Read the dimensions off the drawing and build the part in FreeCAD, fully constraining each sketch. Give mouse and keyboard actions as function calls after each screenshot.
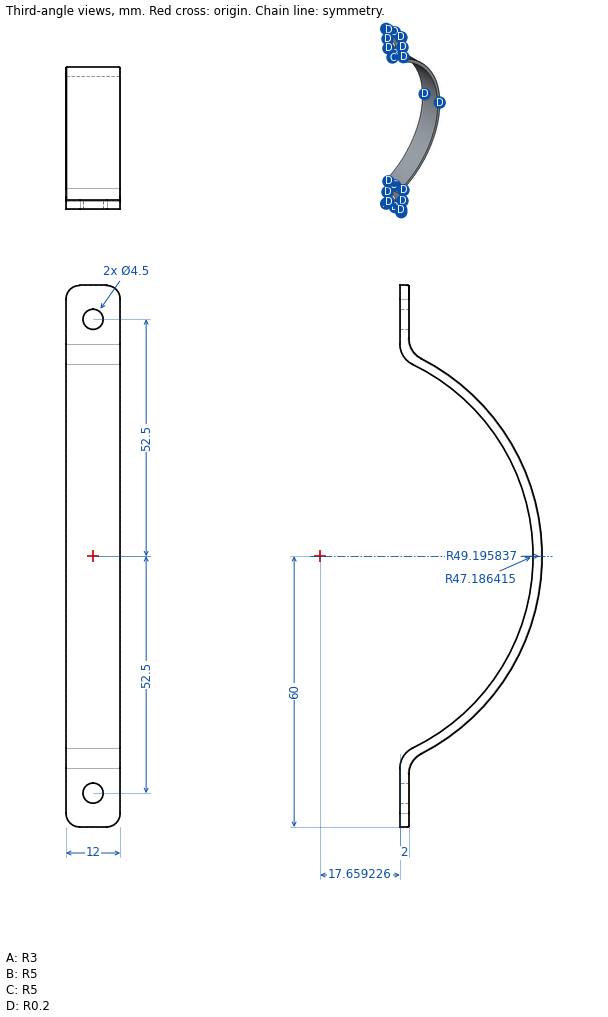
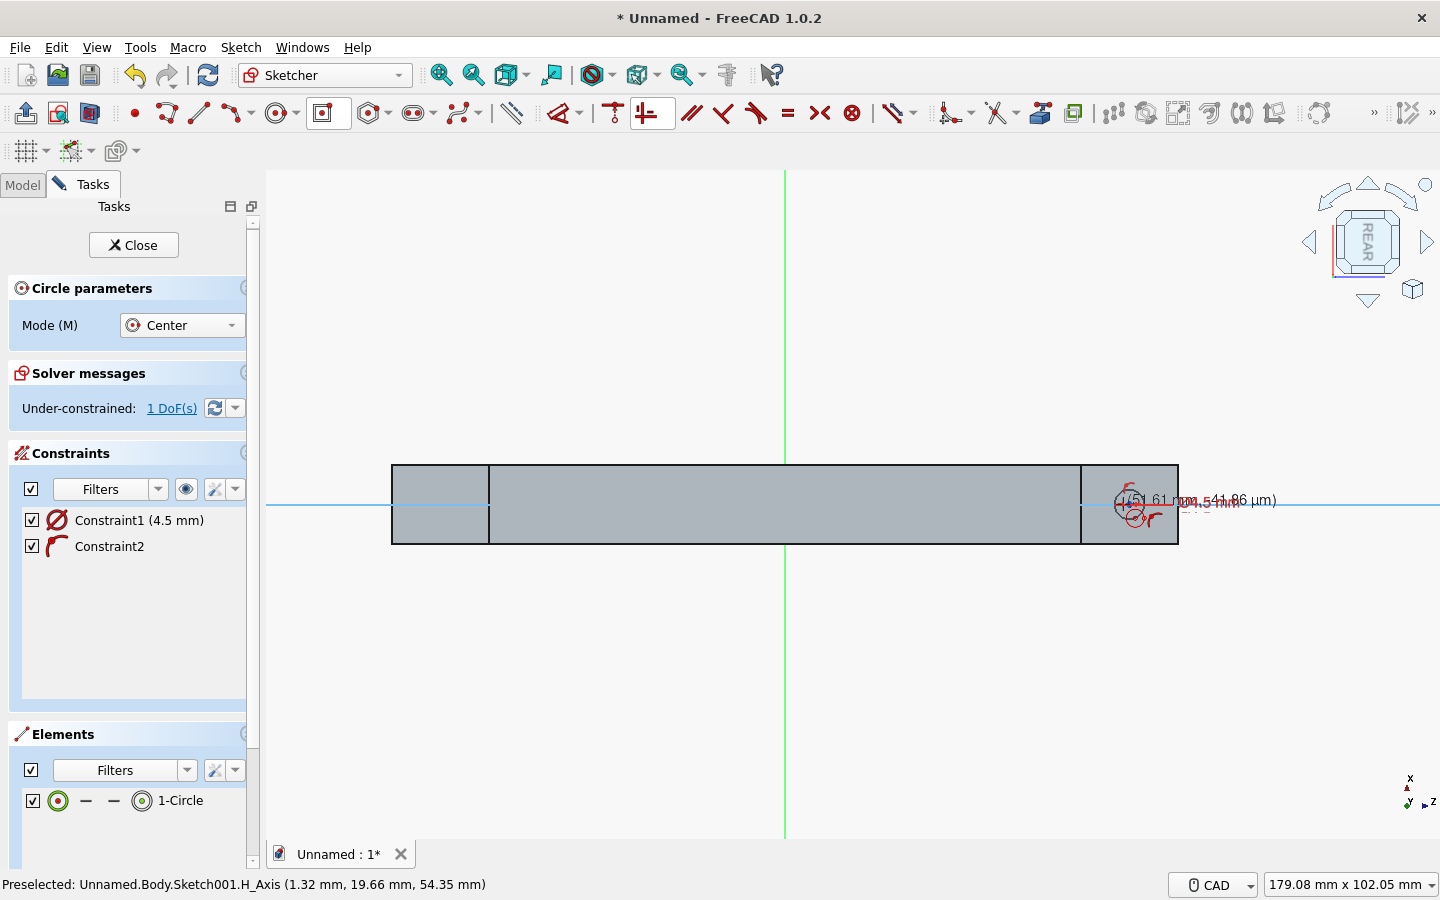
scroll(441, 504, up, 3)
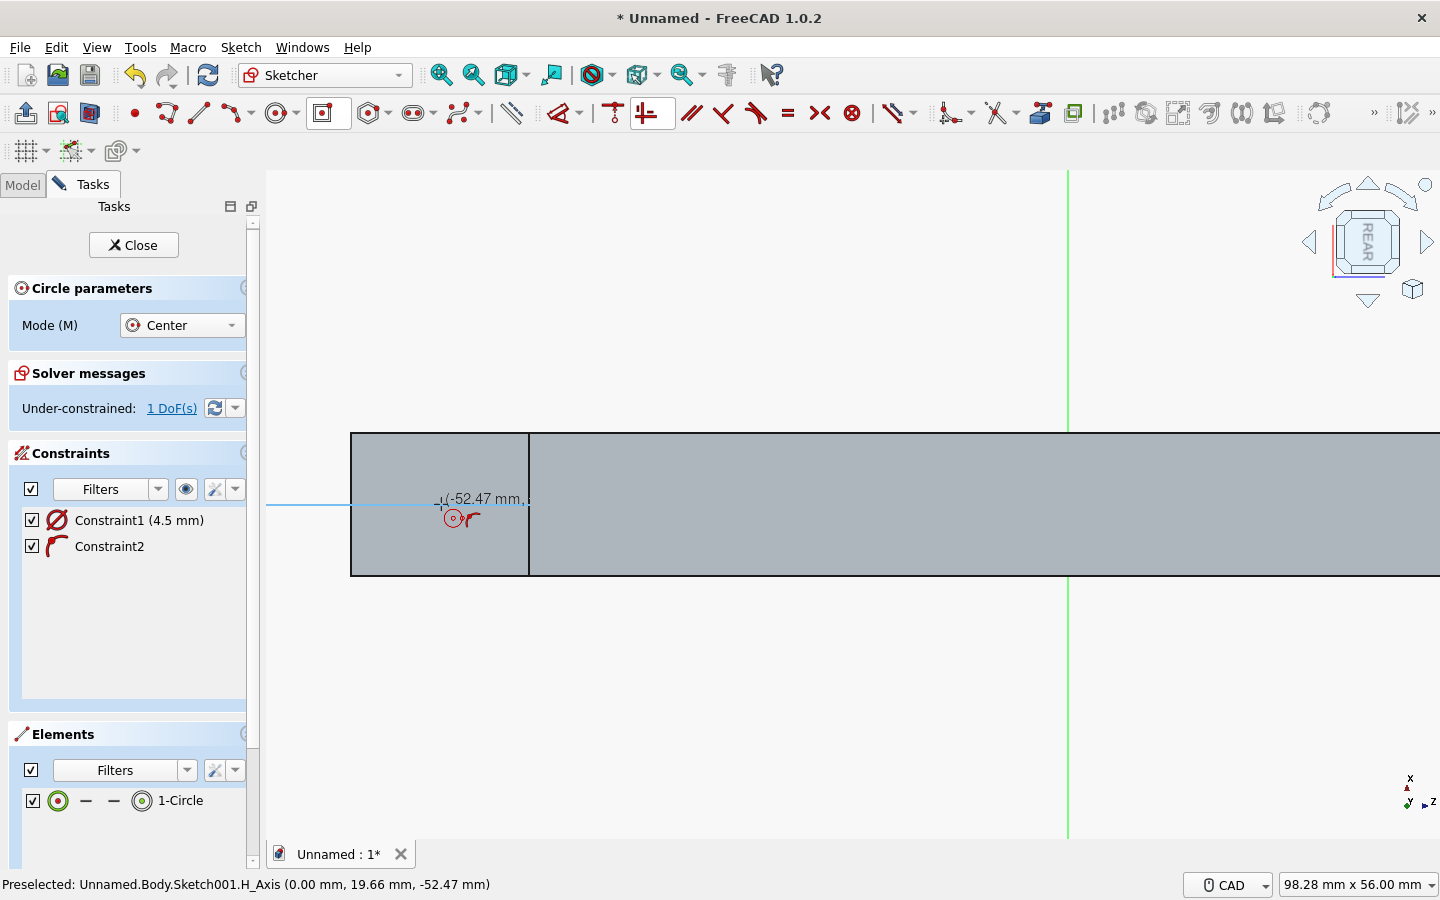
click(441, 504)
move(460, 485)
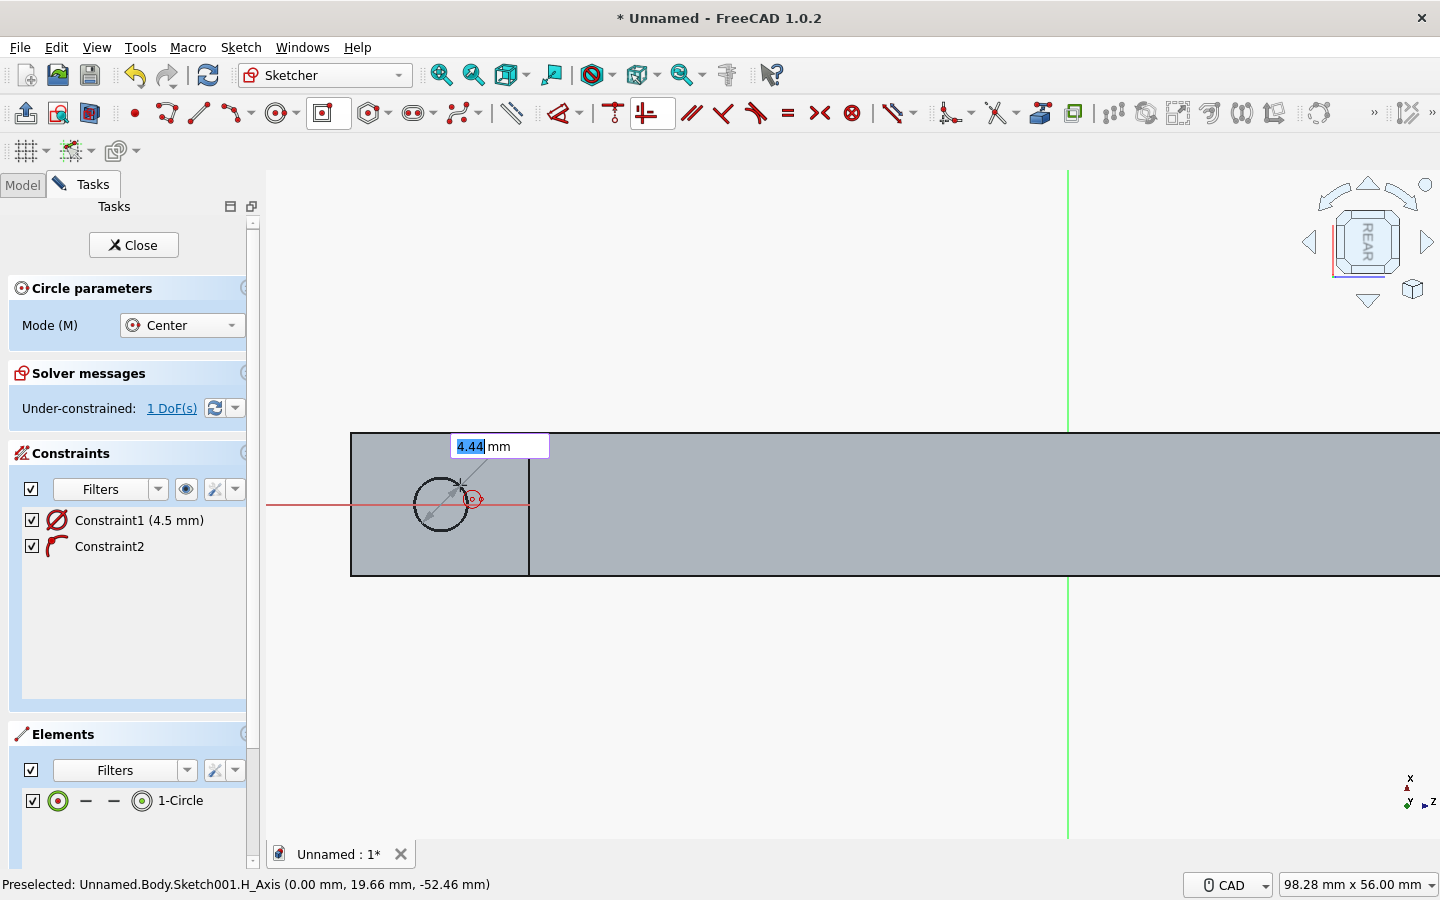
text(4.5)
key(Return)
key(Escape)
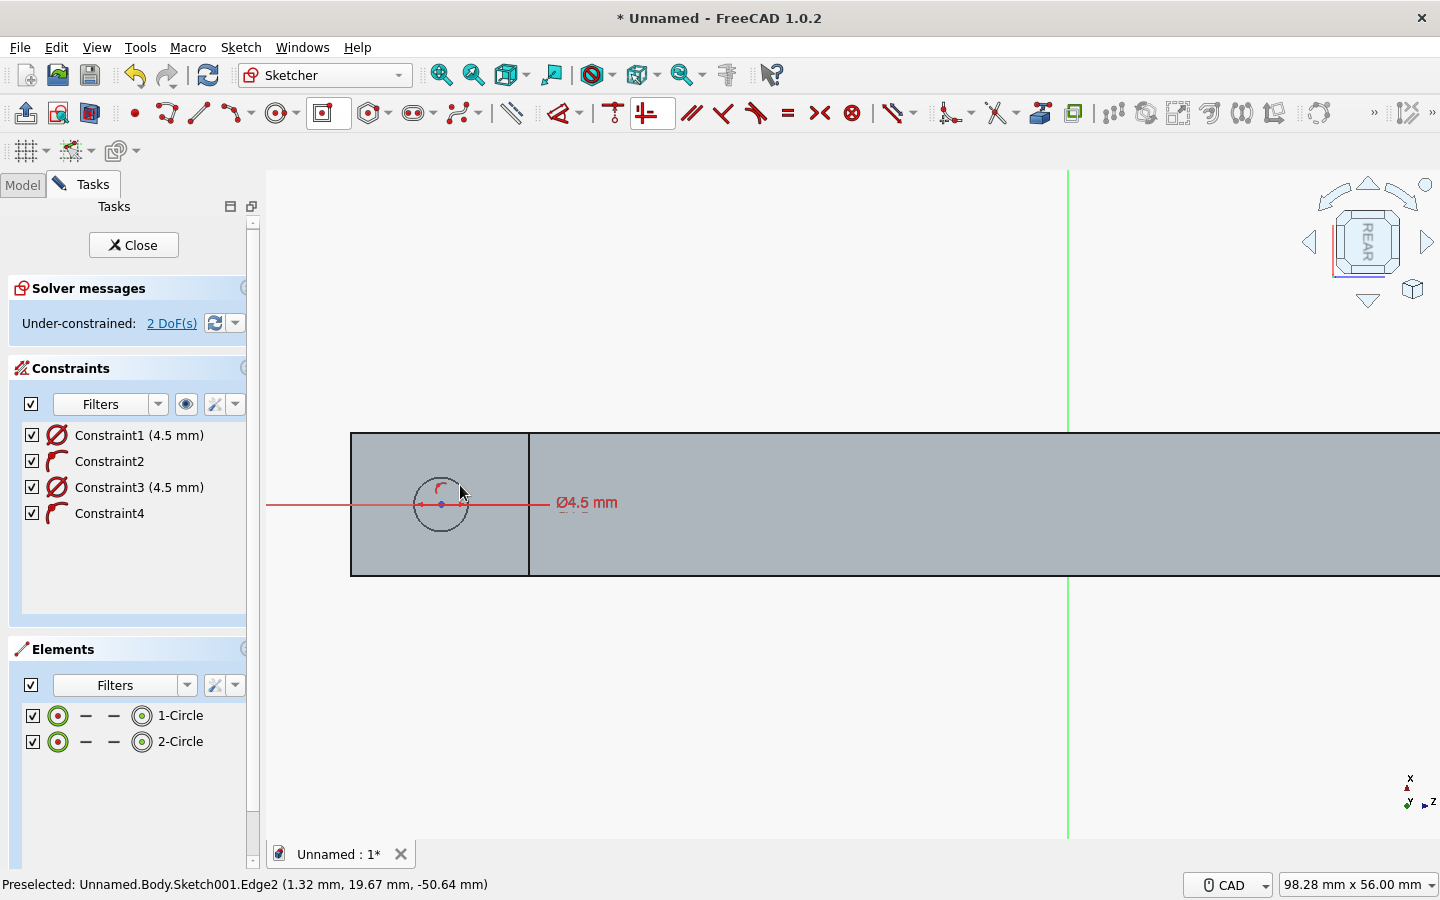
click(558, 114)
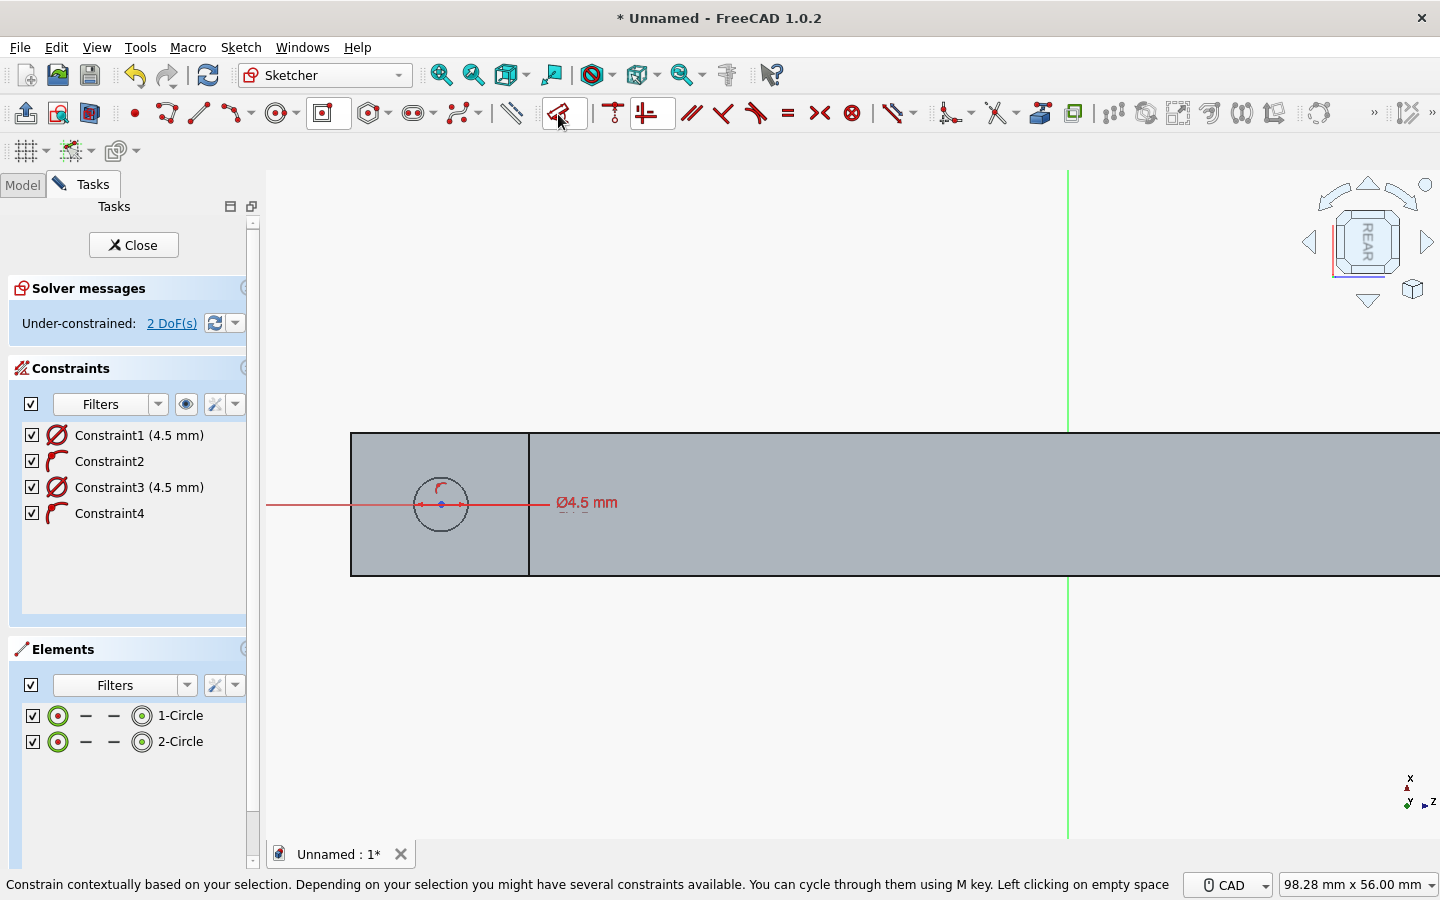
scroll(440, 505, down, 3)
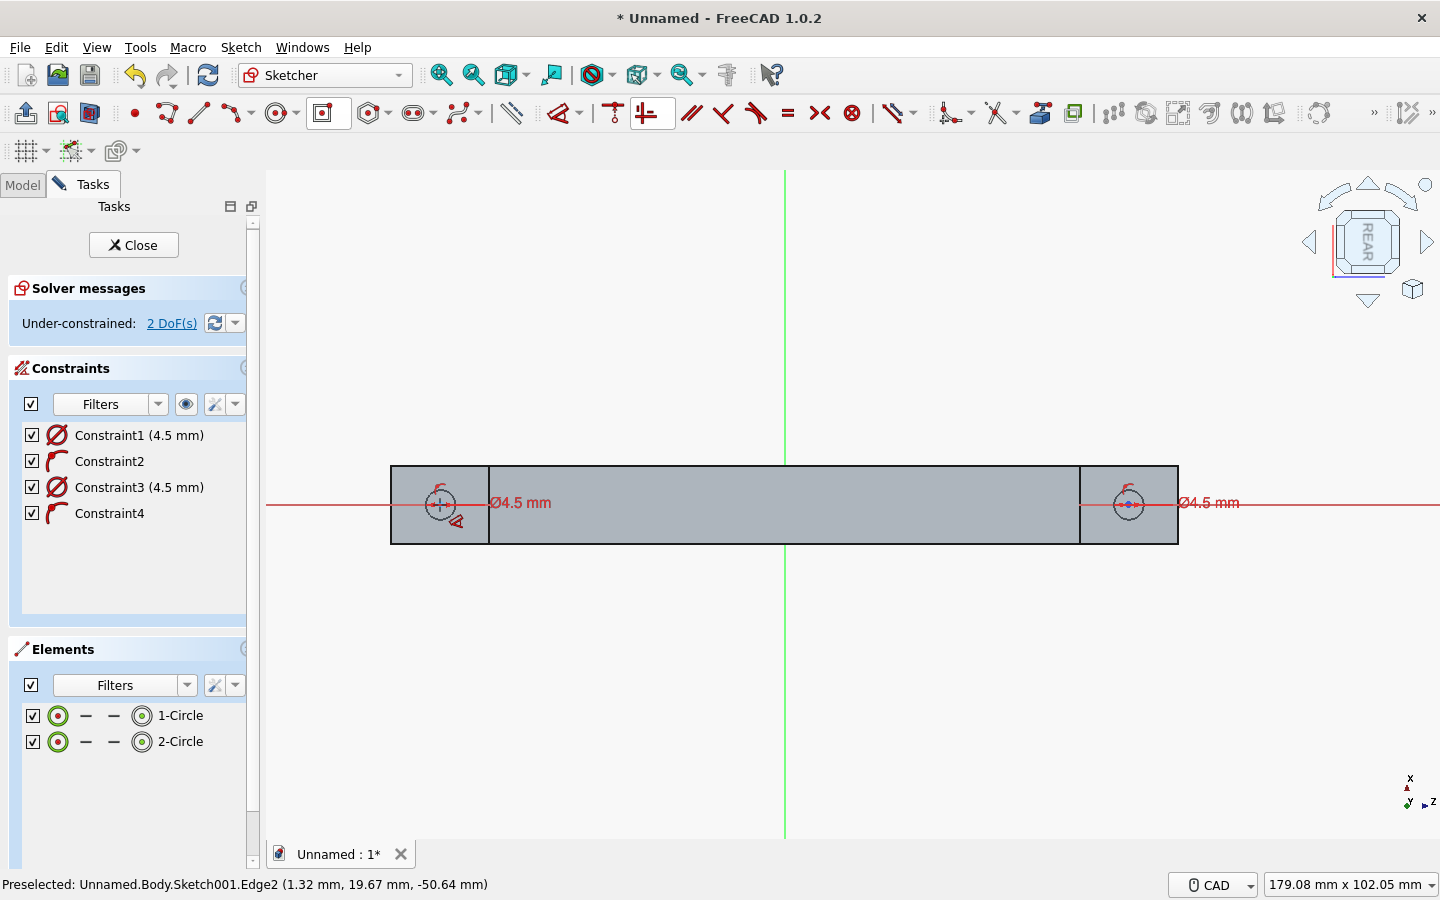
click(1129, 505)
click(957, 539)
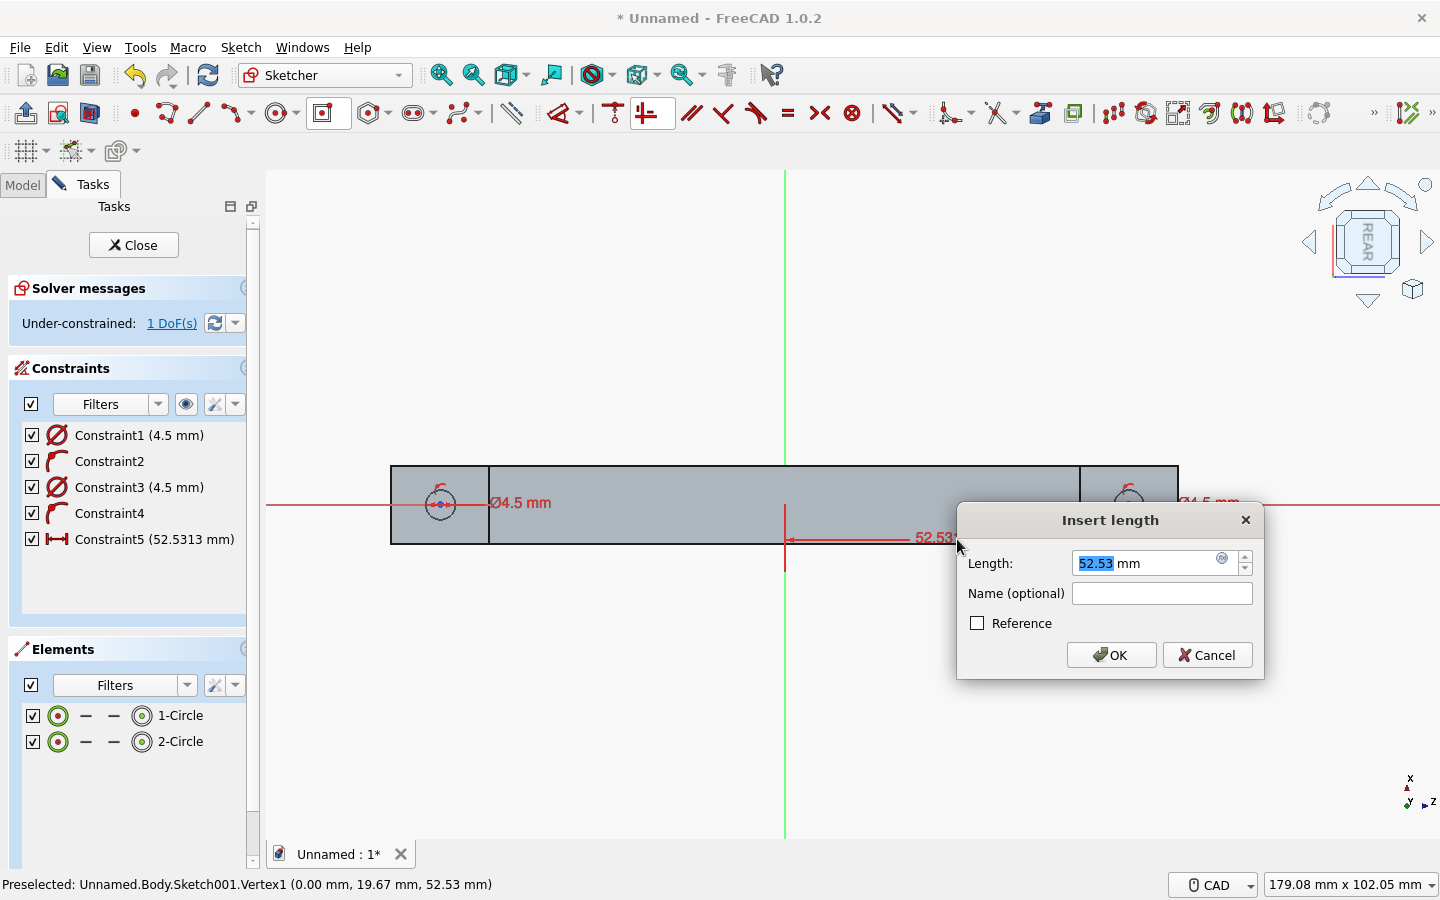
text(52.5)
key(Return)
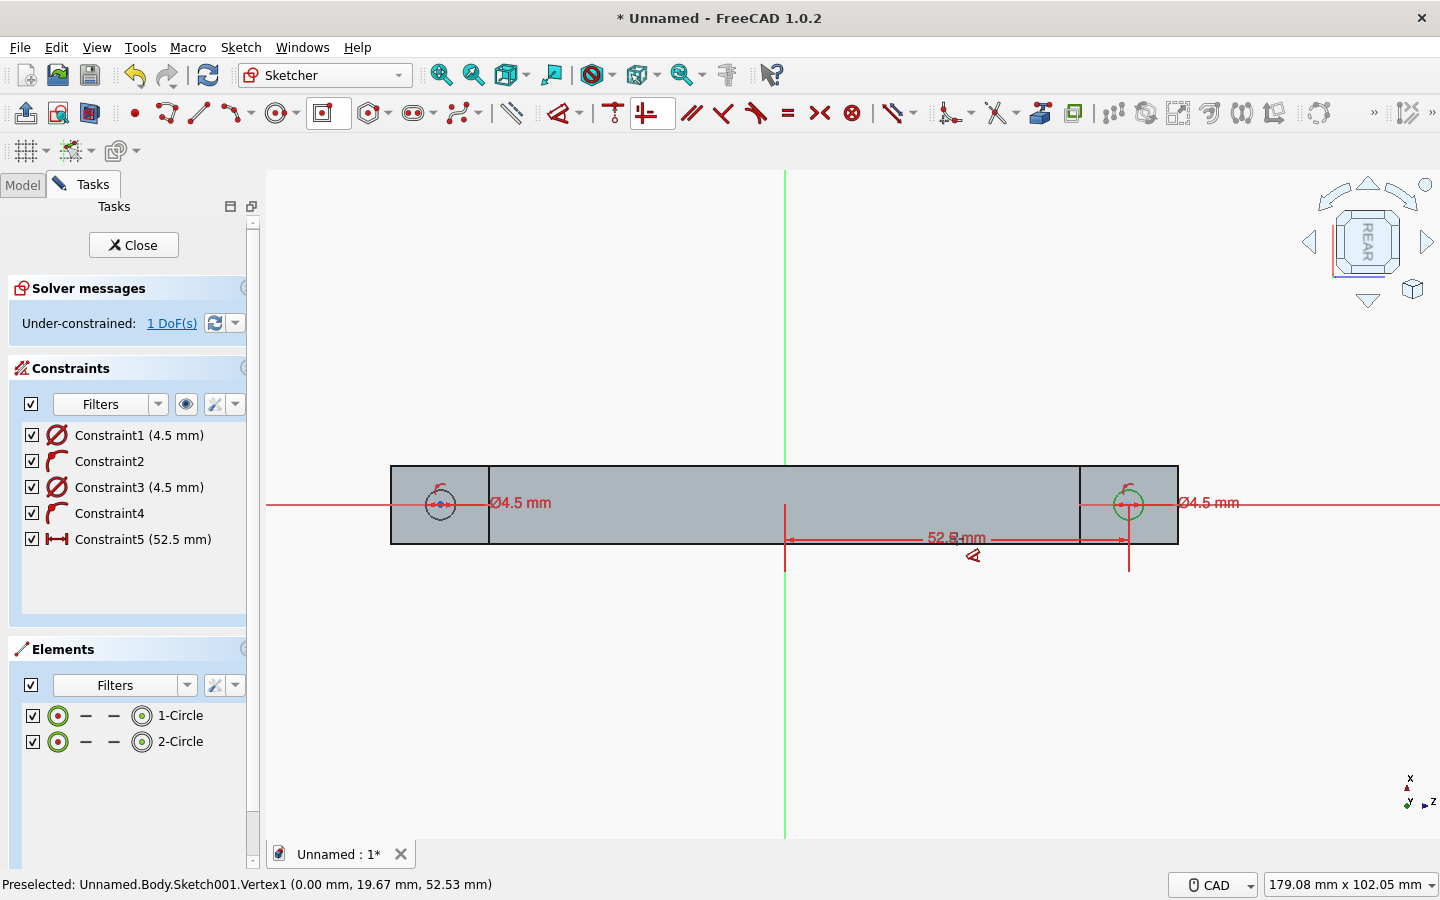
click(441, 505)
click(613, 539)